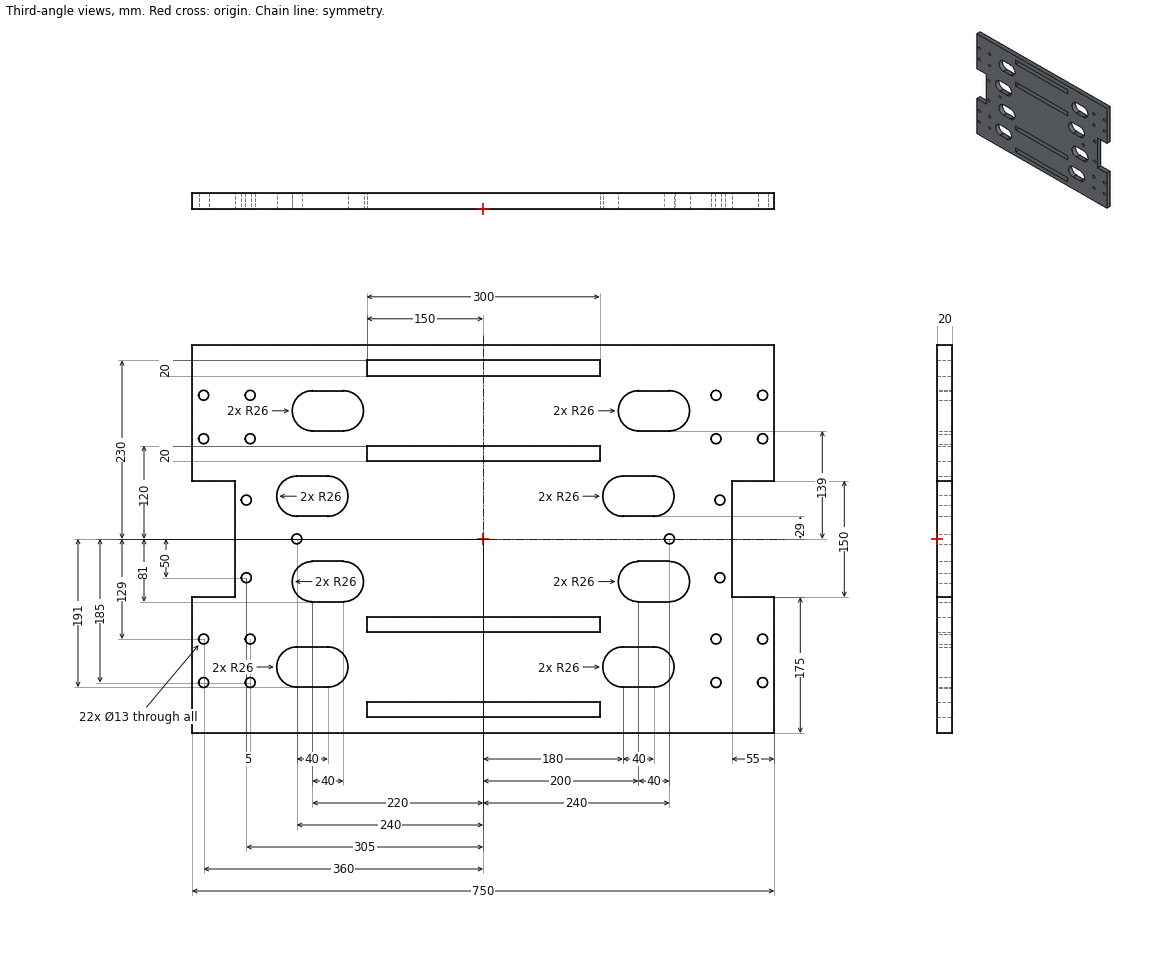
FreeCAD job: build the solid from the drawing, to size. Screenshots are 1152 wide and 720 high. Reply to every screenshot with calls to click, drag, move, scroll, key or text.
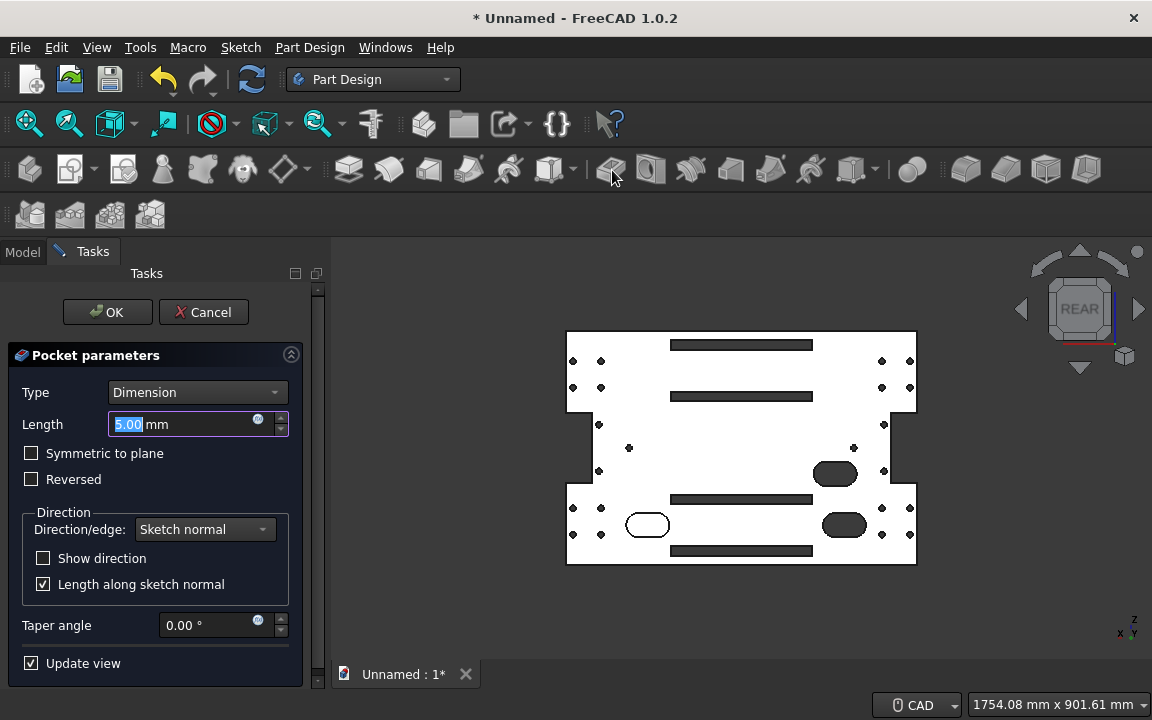
click(198, 392)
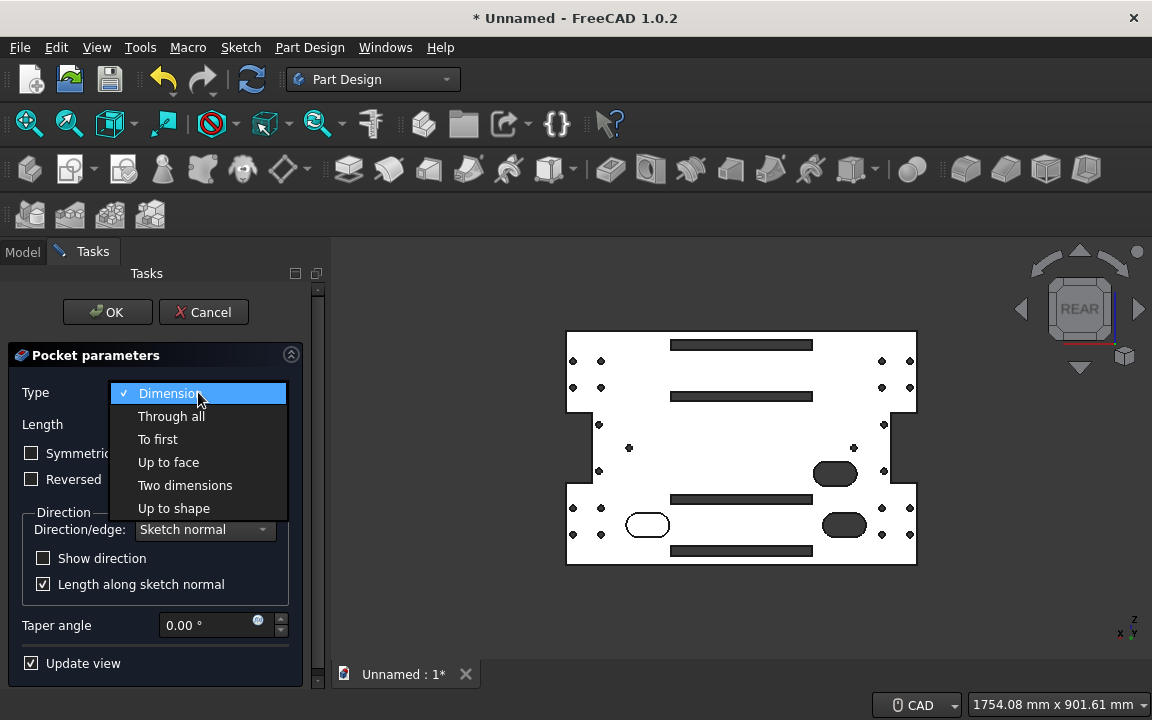
click(198, 440)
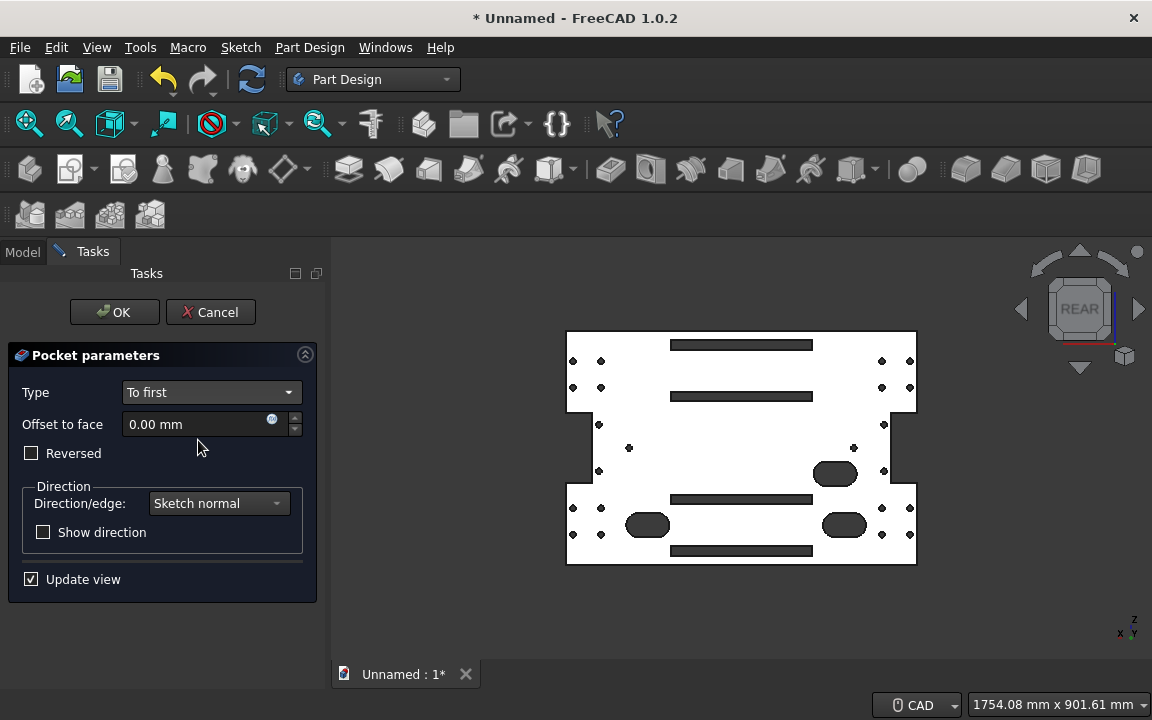
click(115, 312)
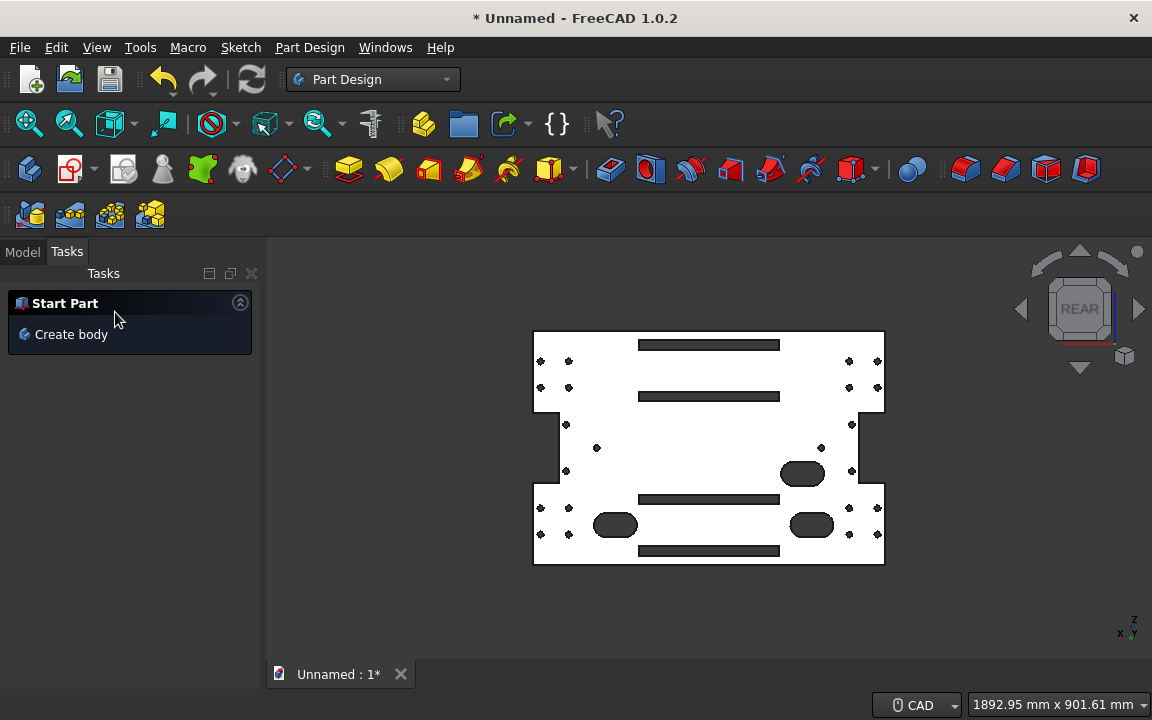
click(659, 447)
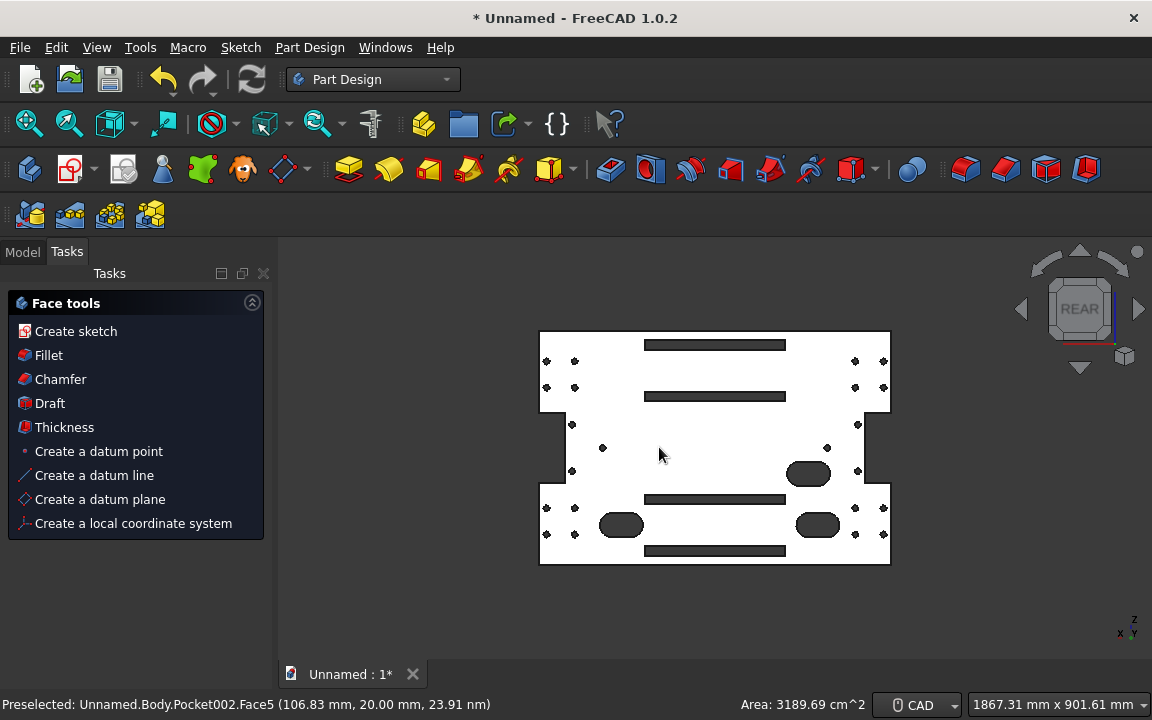
click(70, 170)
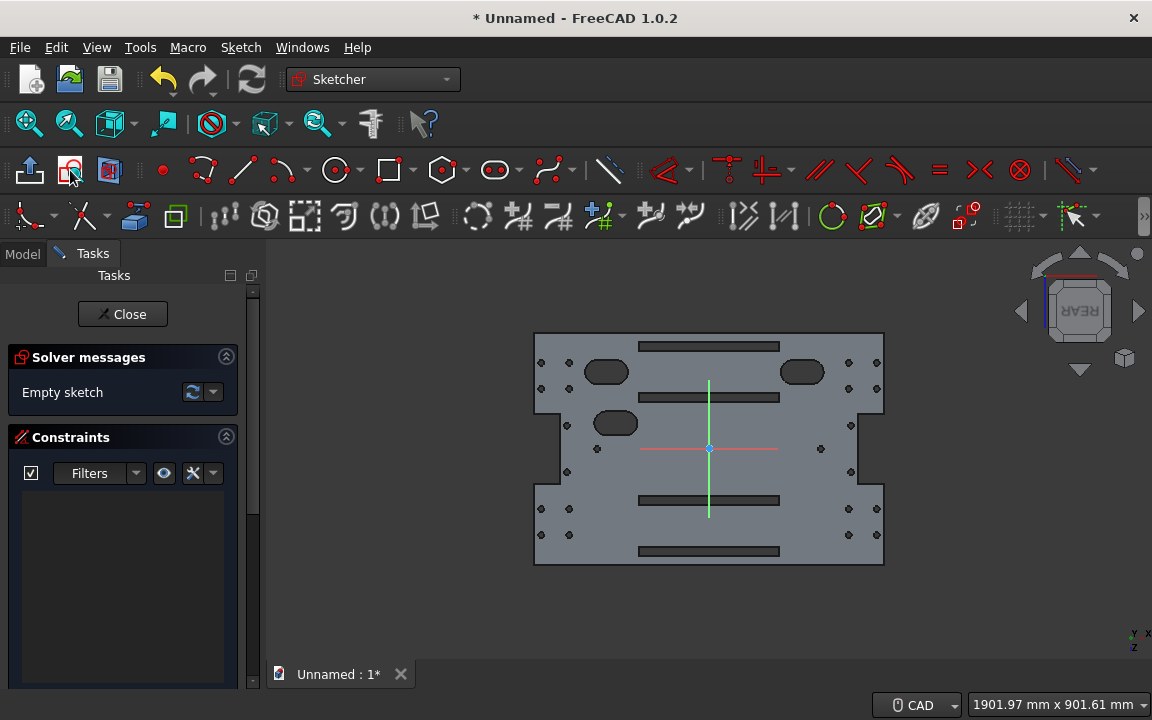
scroll(829, 421, up, 12)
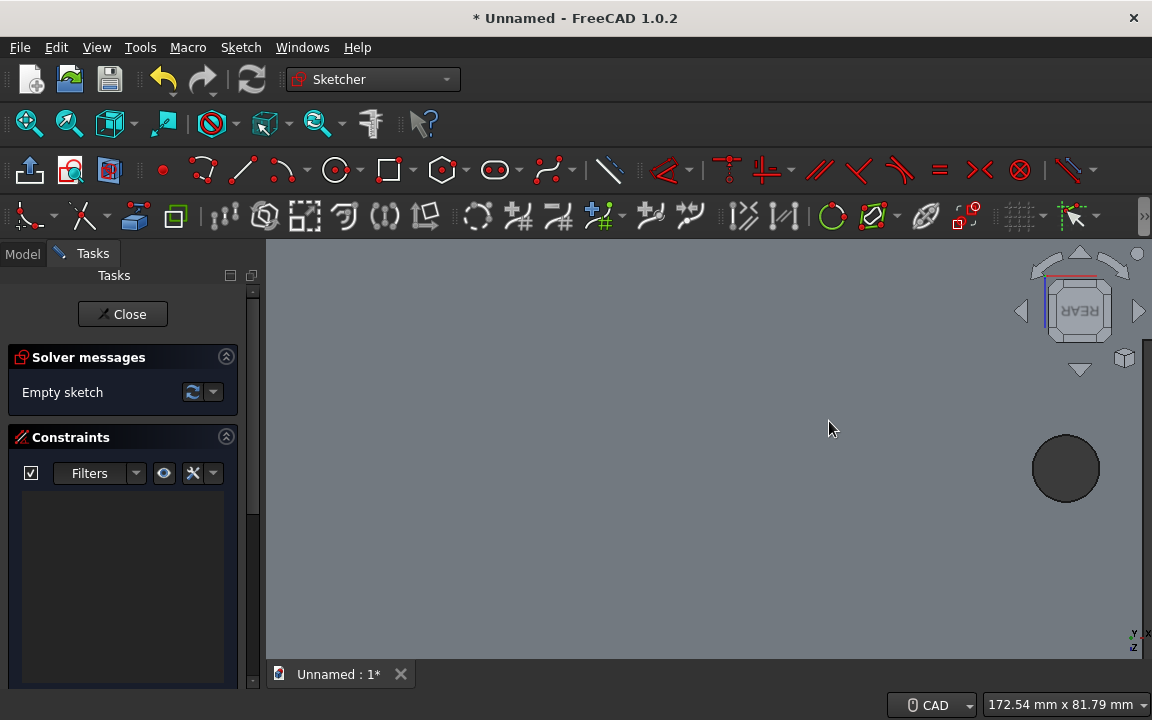
click(496, 170)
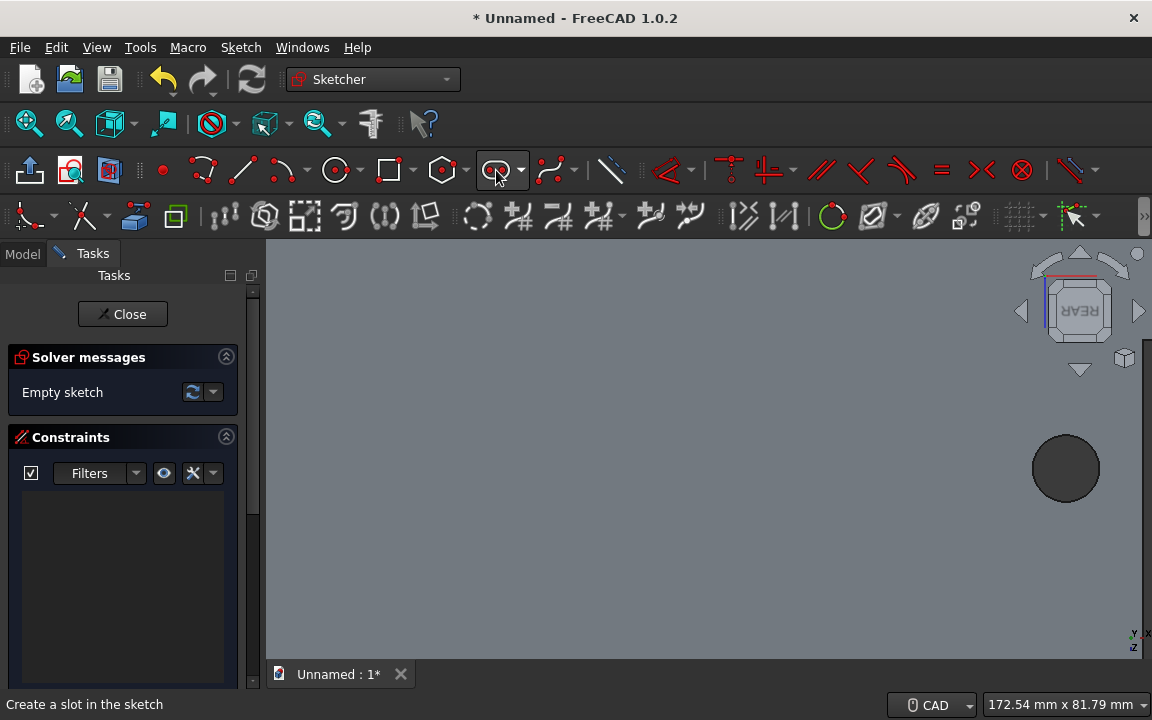
click(527, 443)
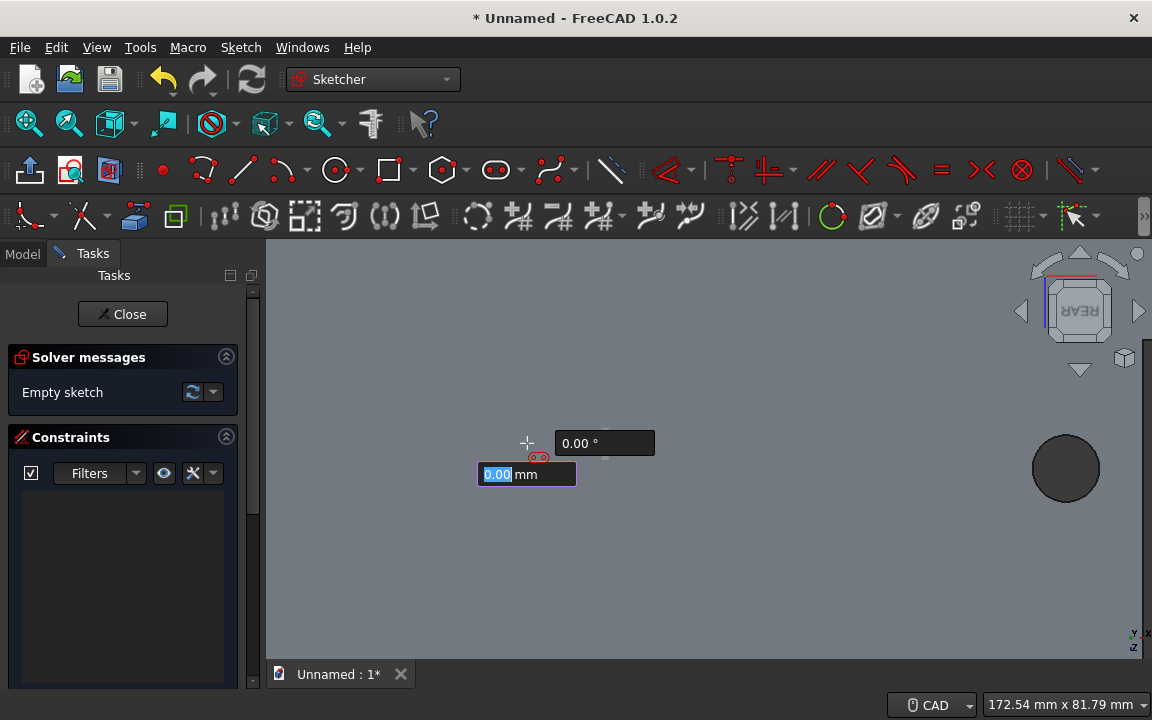
click(732, 443)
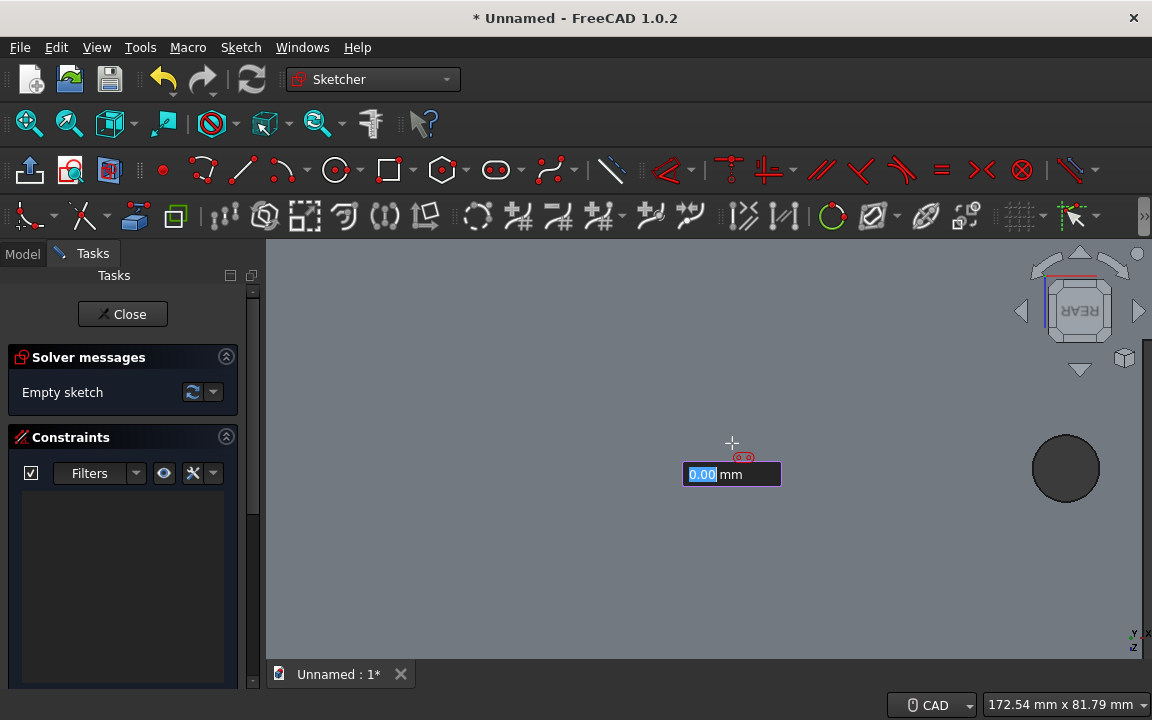
click(630, 309)
key(Escape)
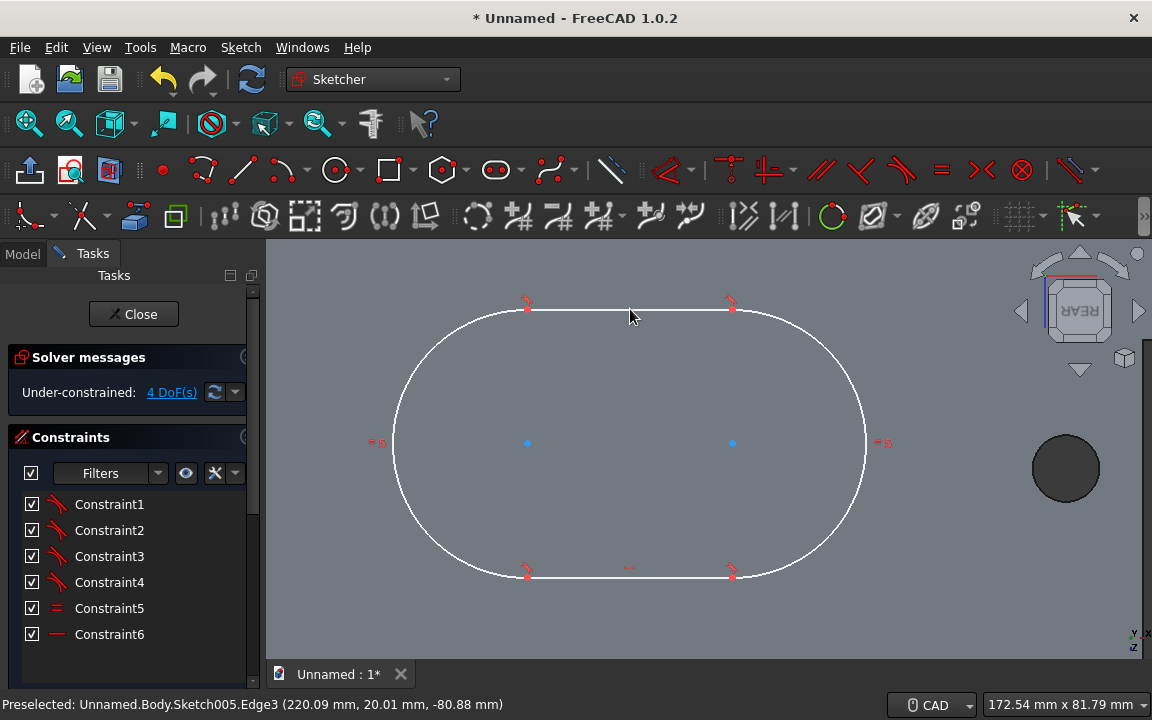
click(666, 170)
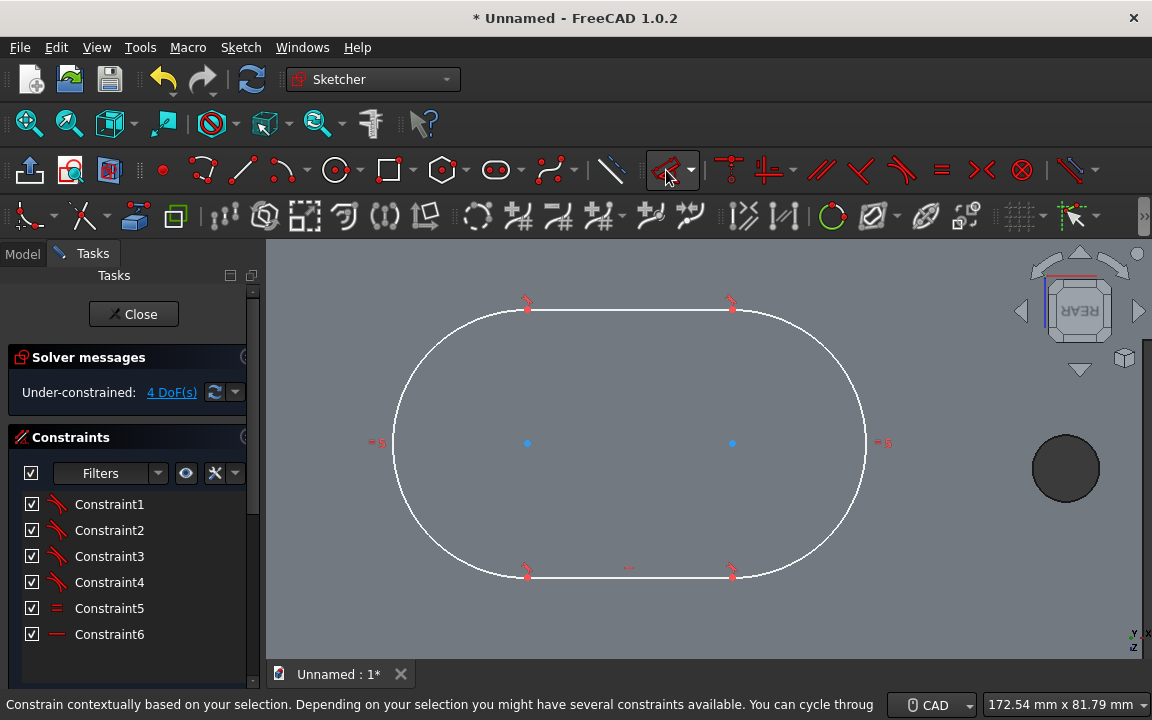
click(419, 365)
click(393, 346)